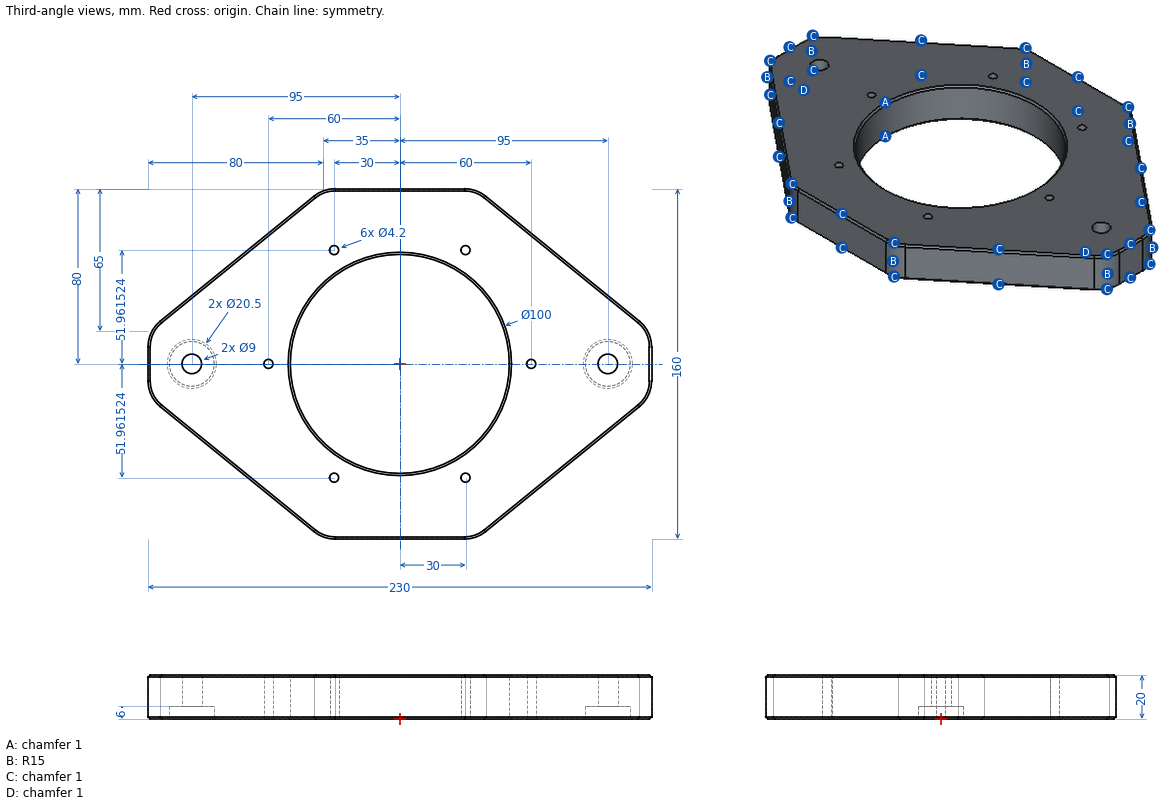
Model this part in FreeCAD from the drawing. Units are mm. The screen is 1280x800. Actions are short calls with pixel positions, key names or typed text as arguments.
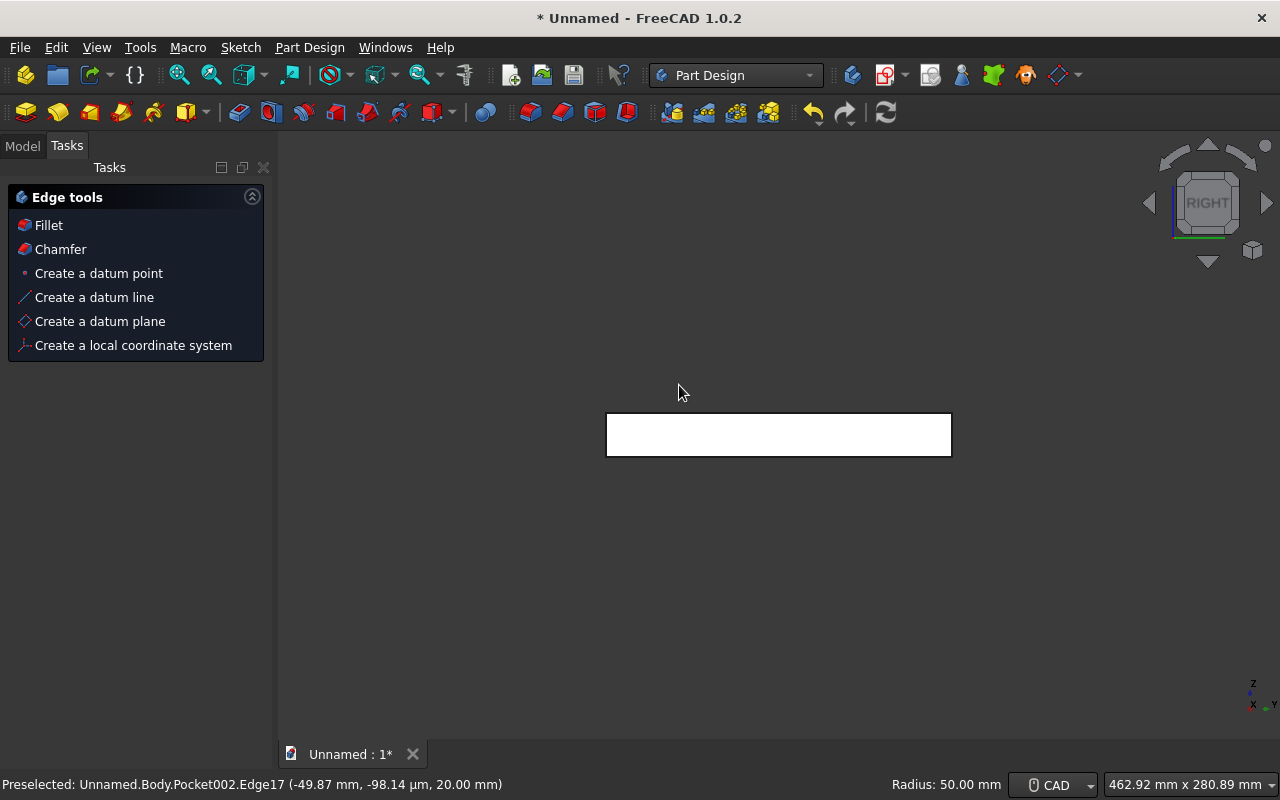
click(180, 76)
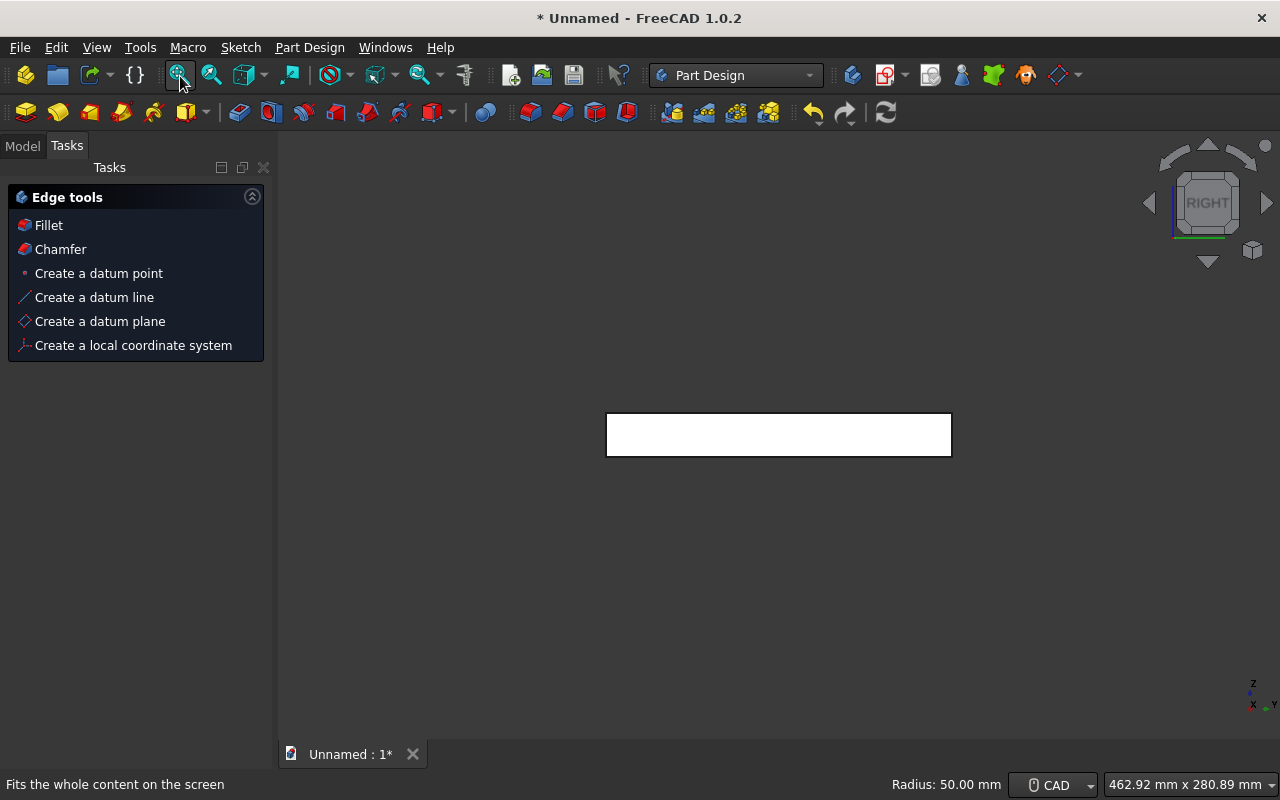
key(5)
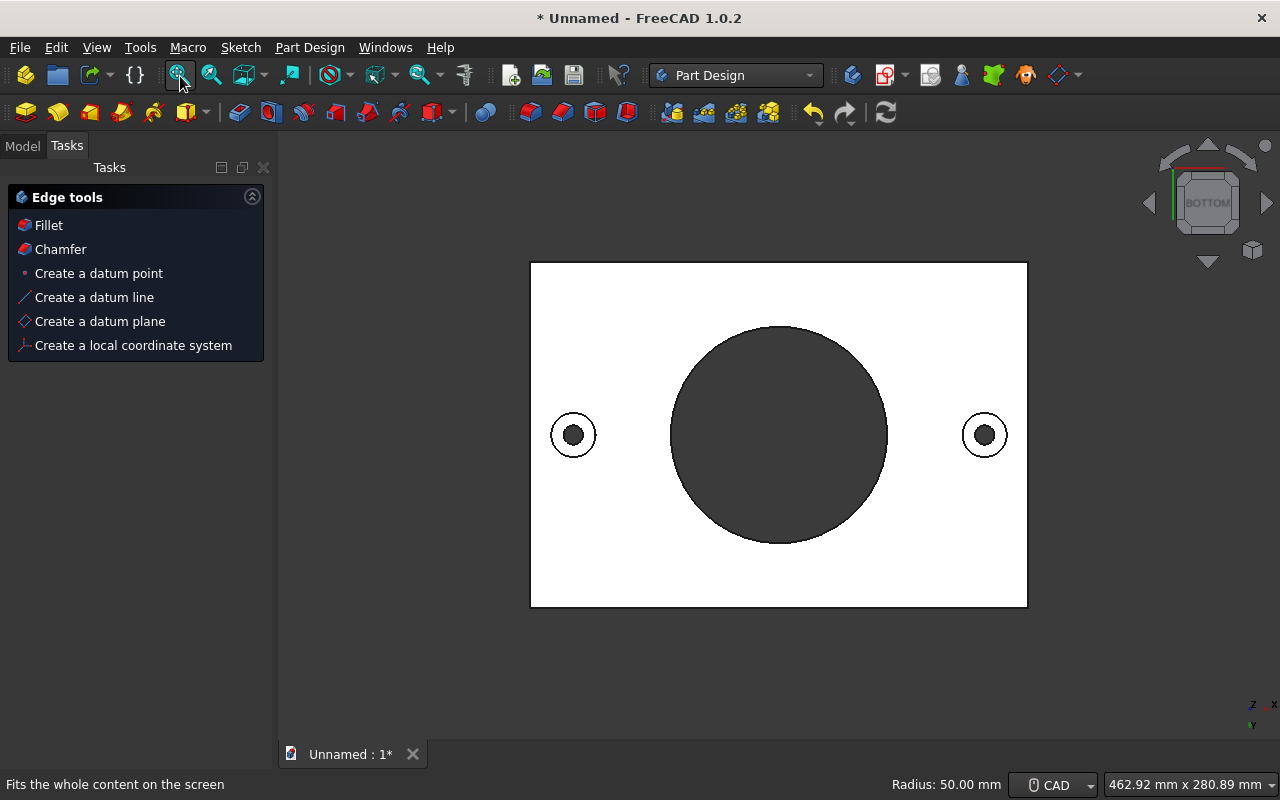
click(671, 434, ctrl)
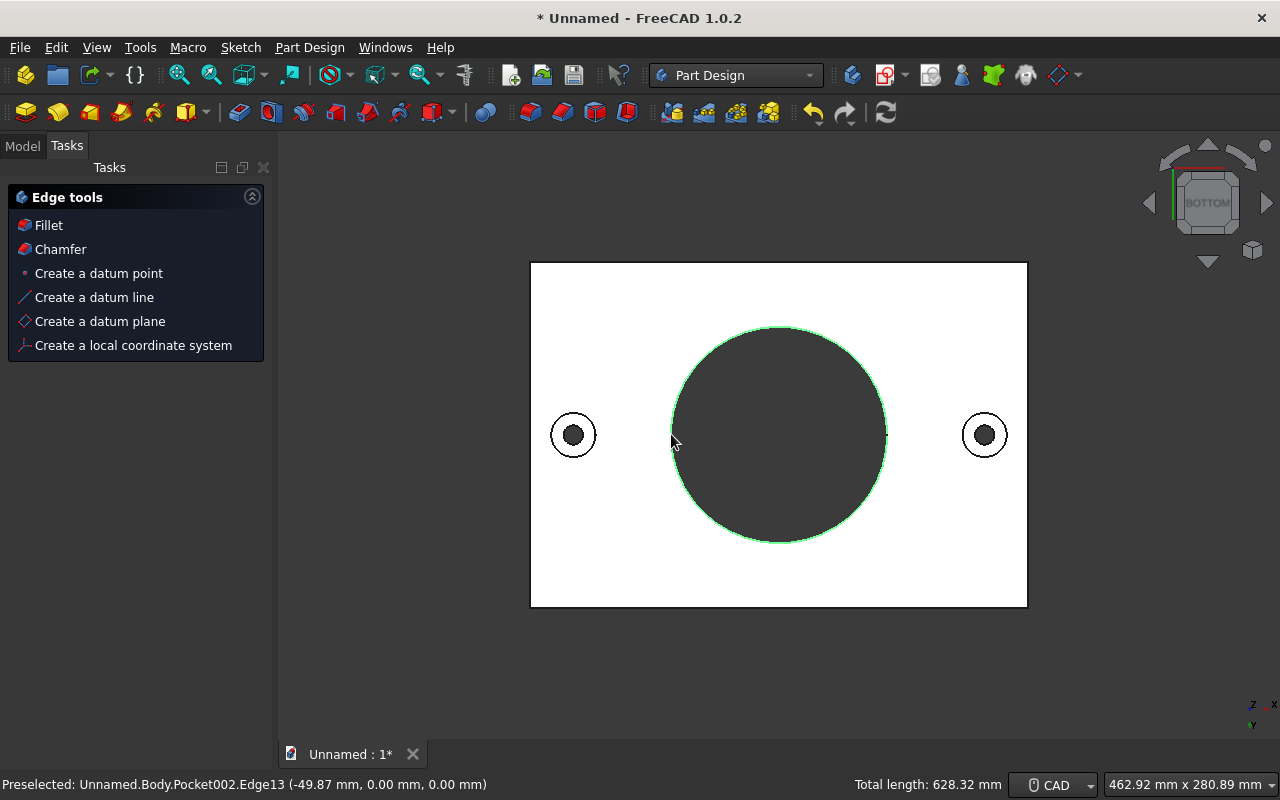
click(564, 112)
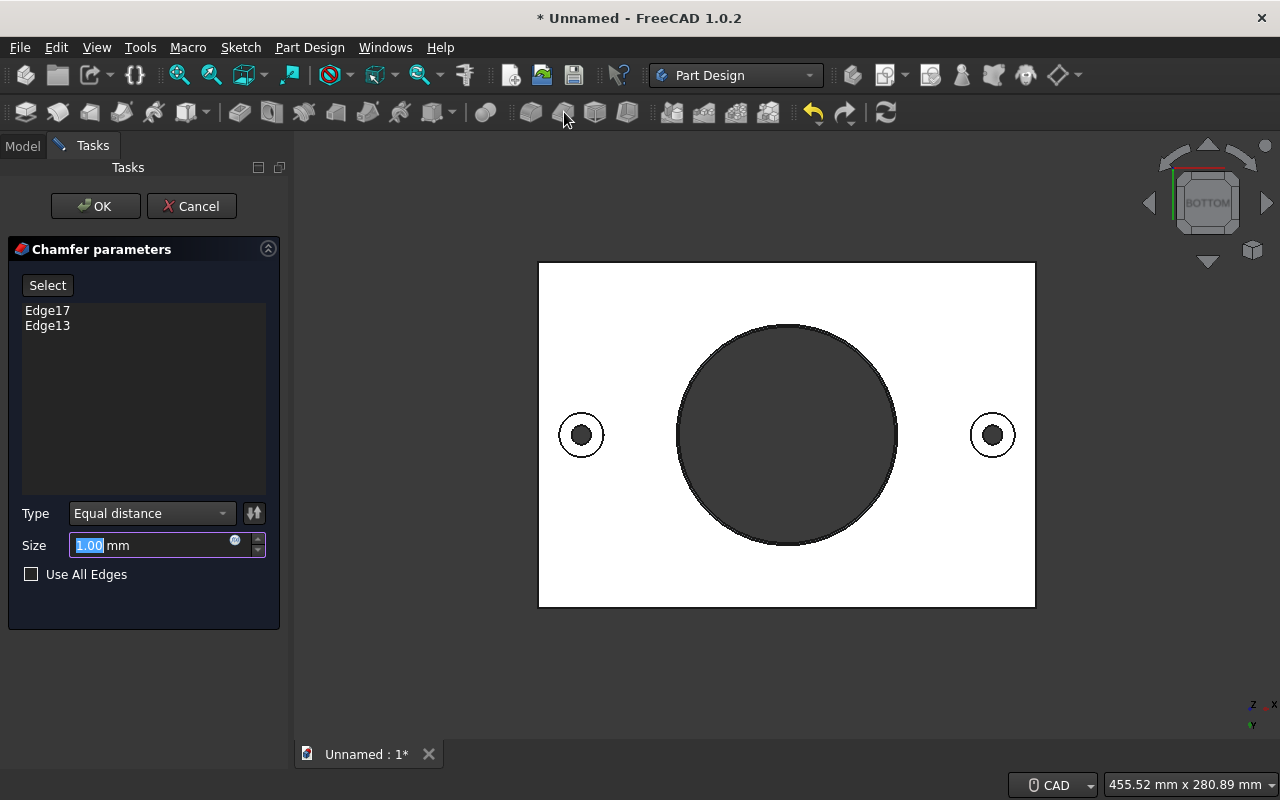
text(1)
key(Tab)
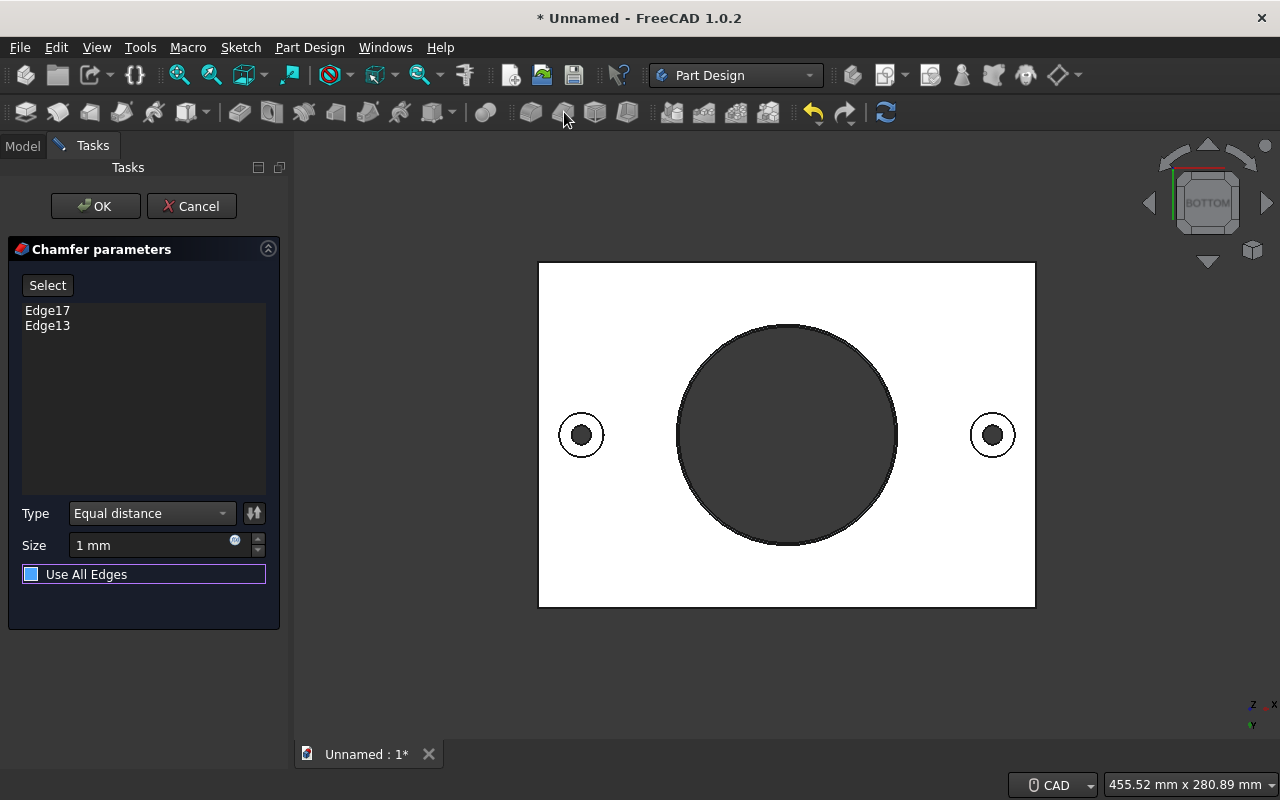
click(96, 206)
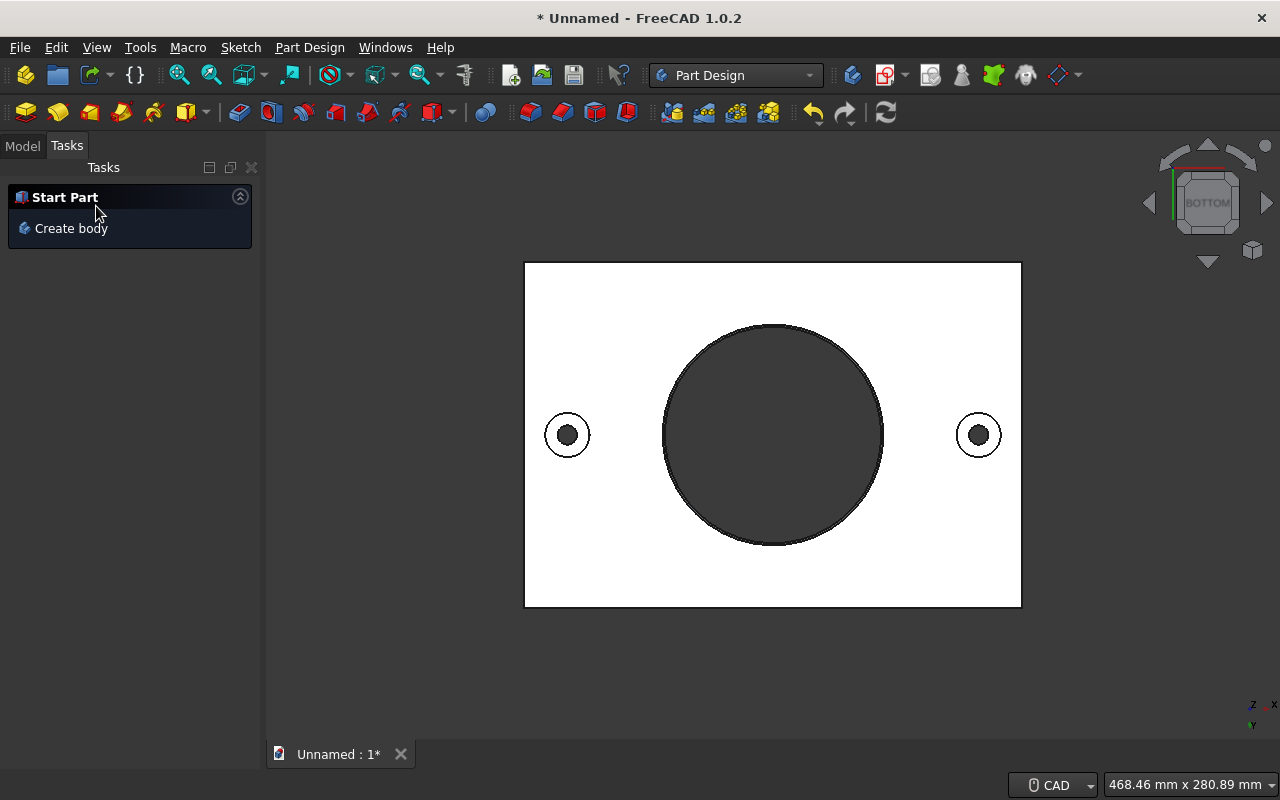
key(0)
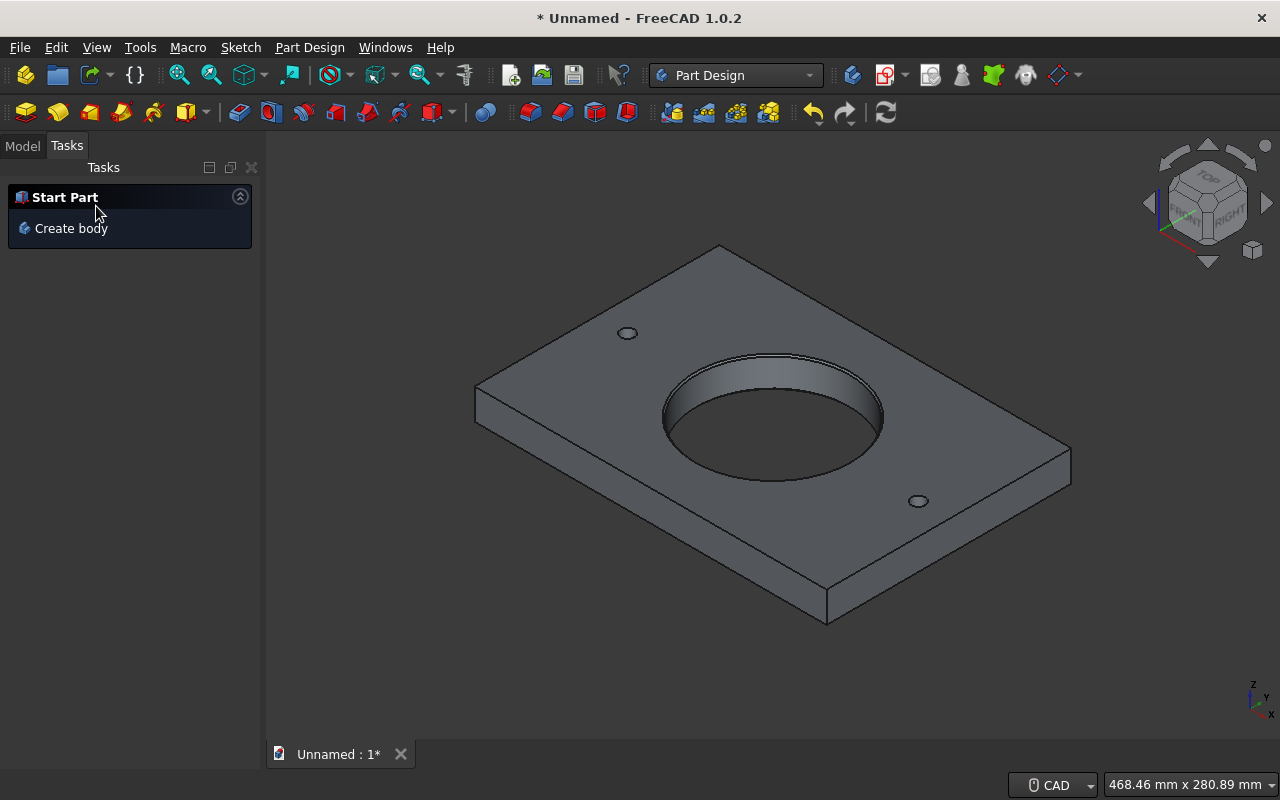
click(944, 434)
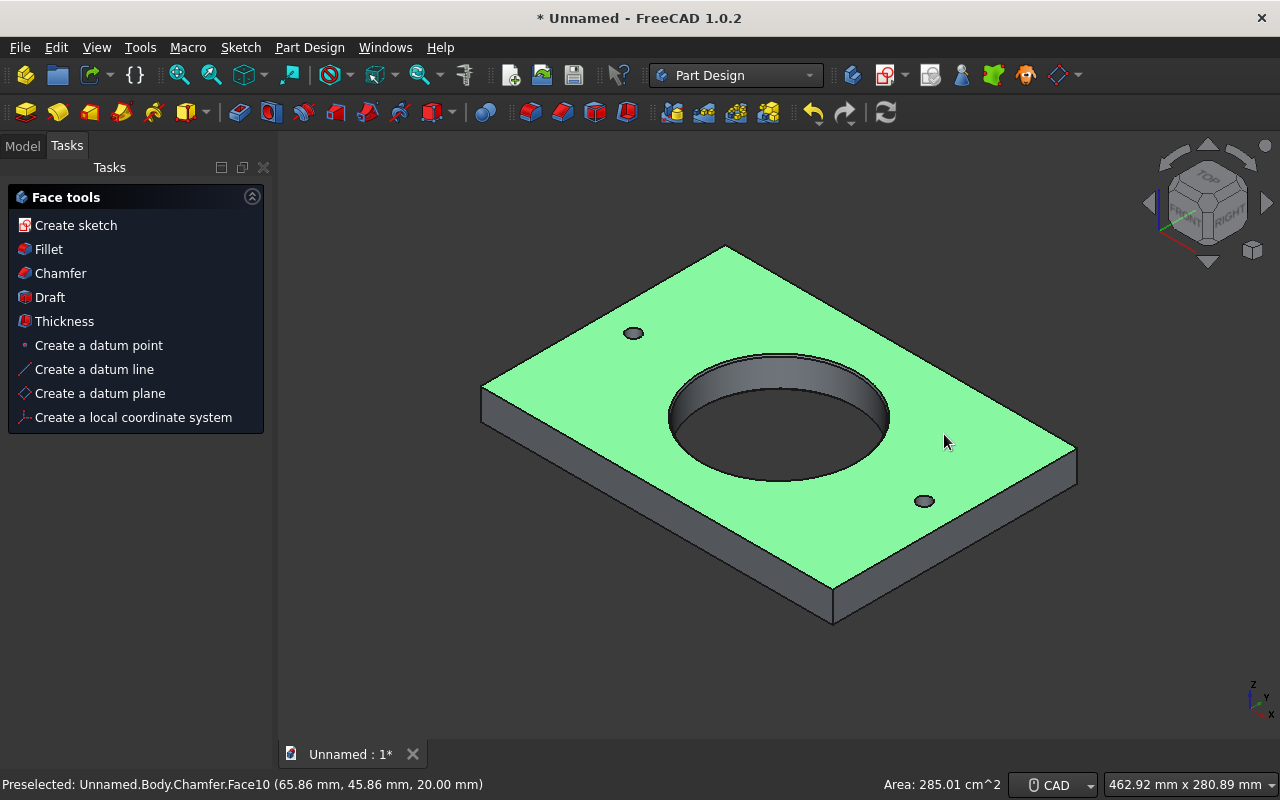
click(886, 76)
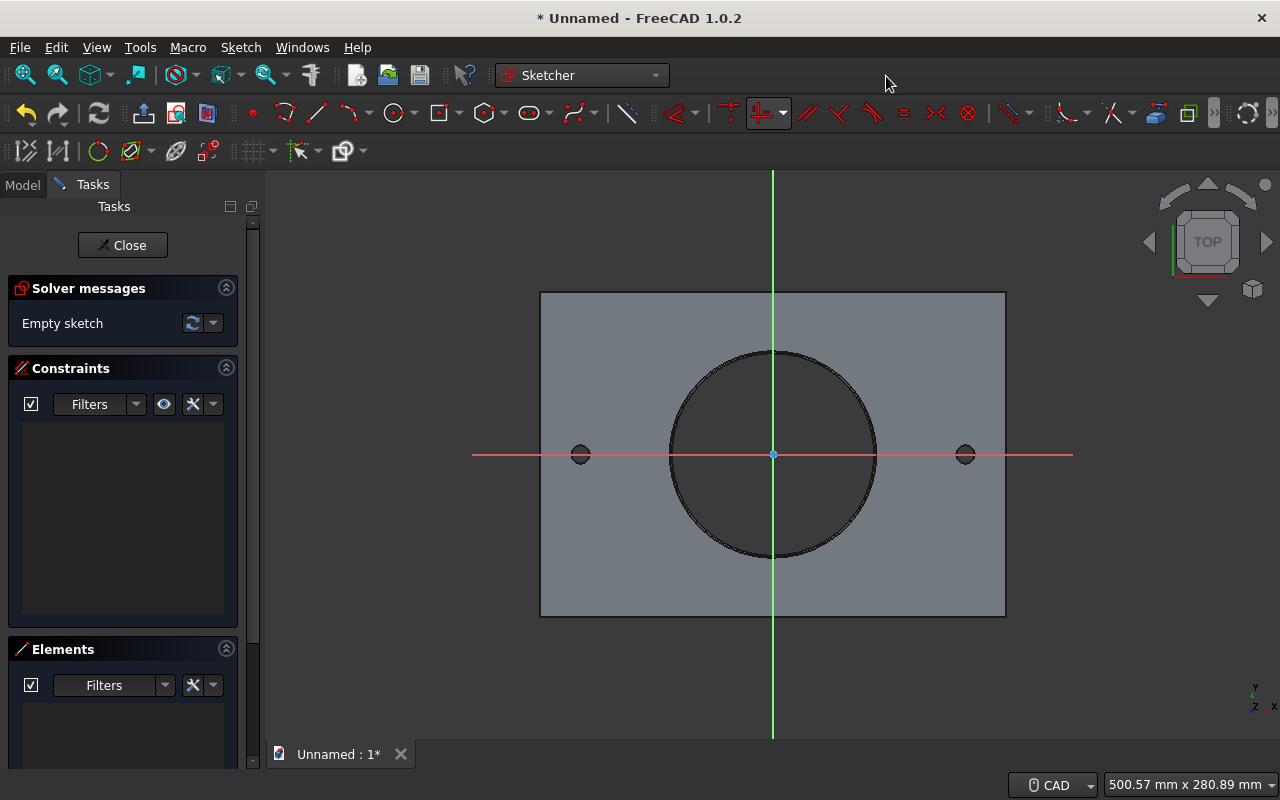
click(286, 114)